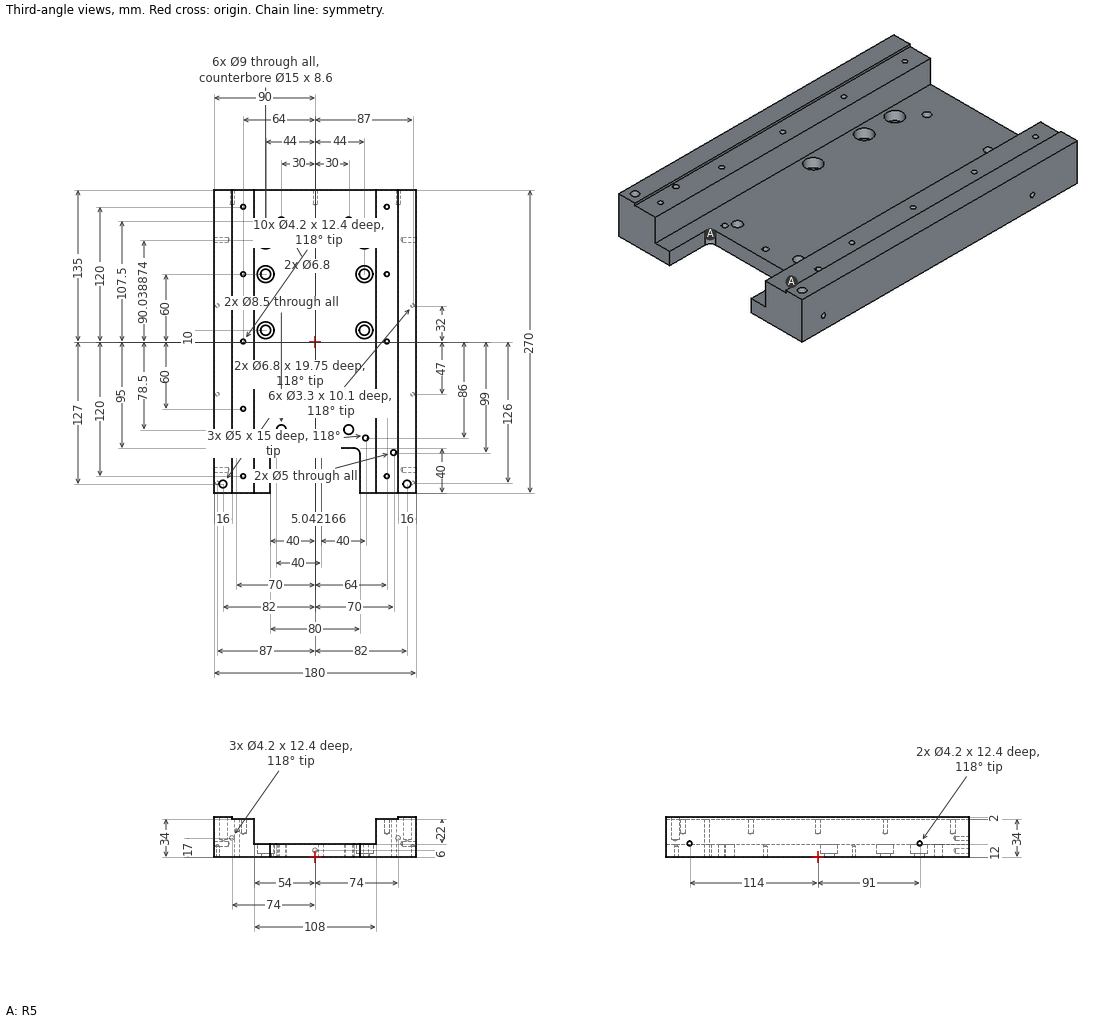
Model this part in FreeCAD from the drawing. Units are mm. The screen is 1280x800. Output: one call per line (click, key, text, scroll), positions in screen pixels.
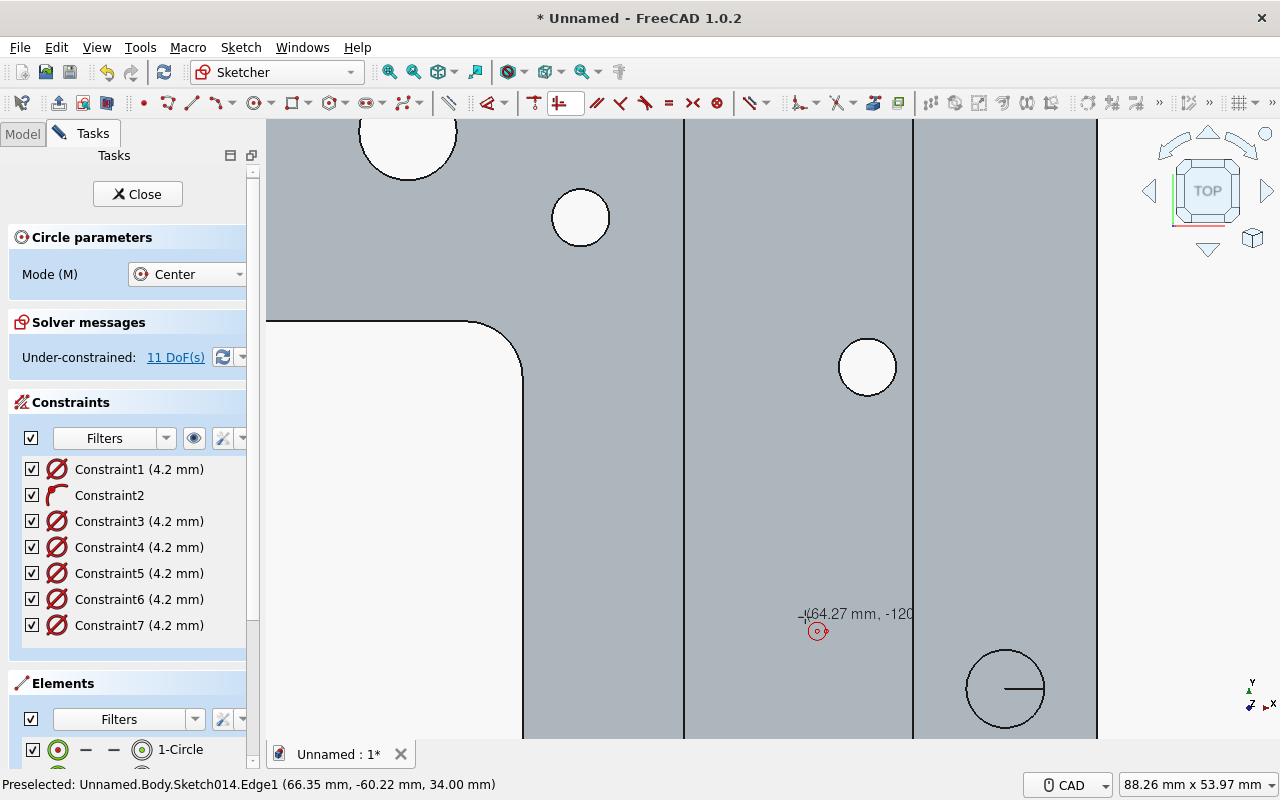
scroll(805, 617, down, 10)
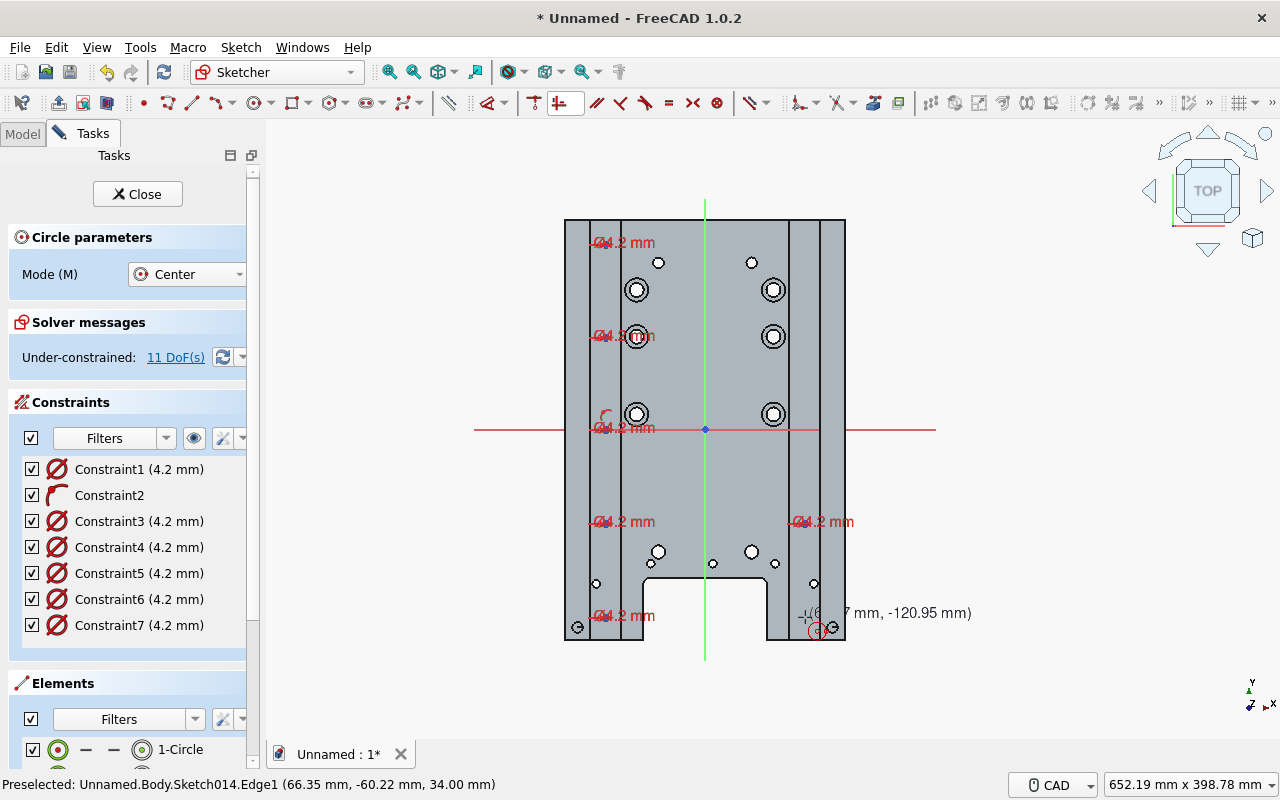
click(805, 617)
move(807, 614)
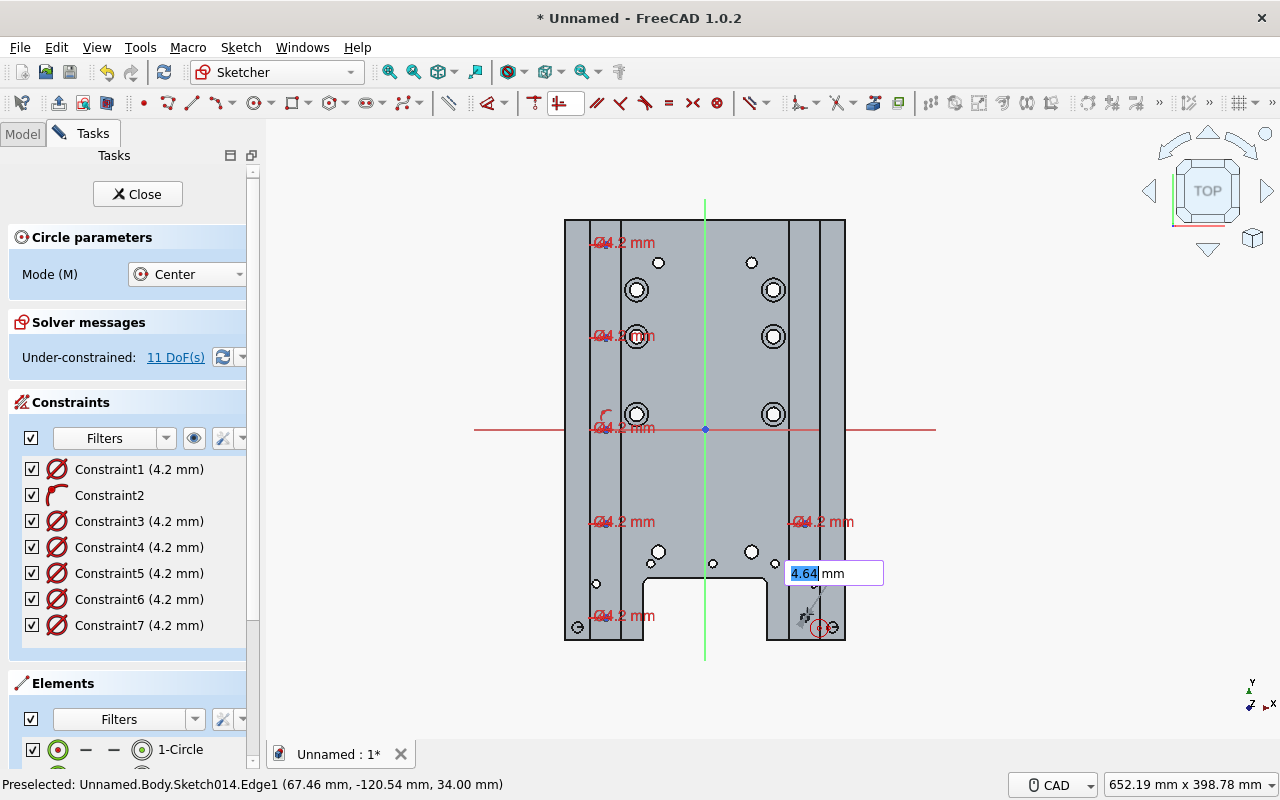
text(4.2)
key(Return)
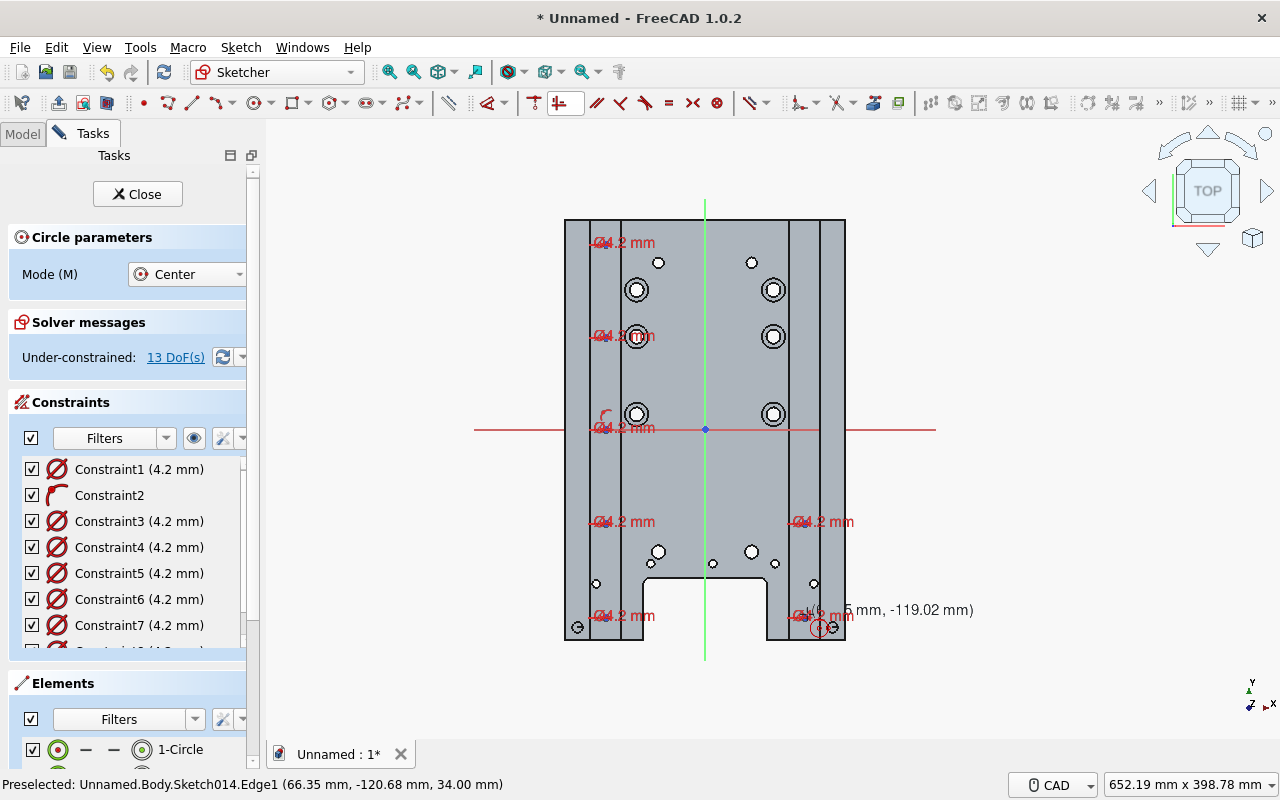
scroll(805, 243, up, 10)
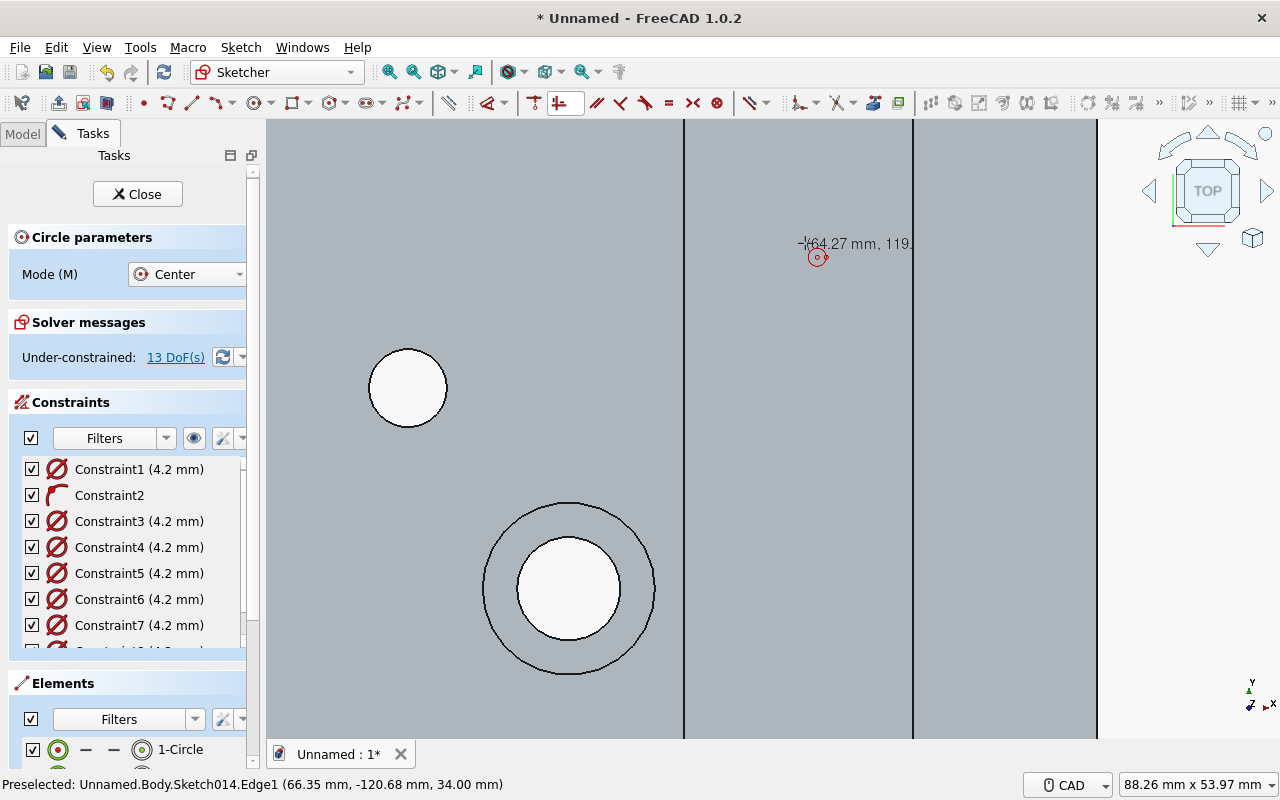
scroll(805, 242, down, 10)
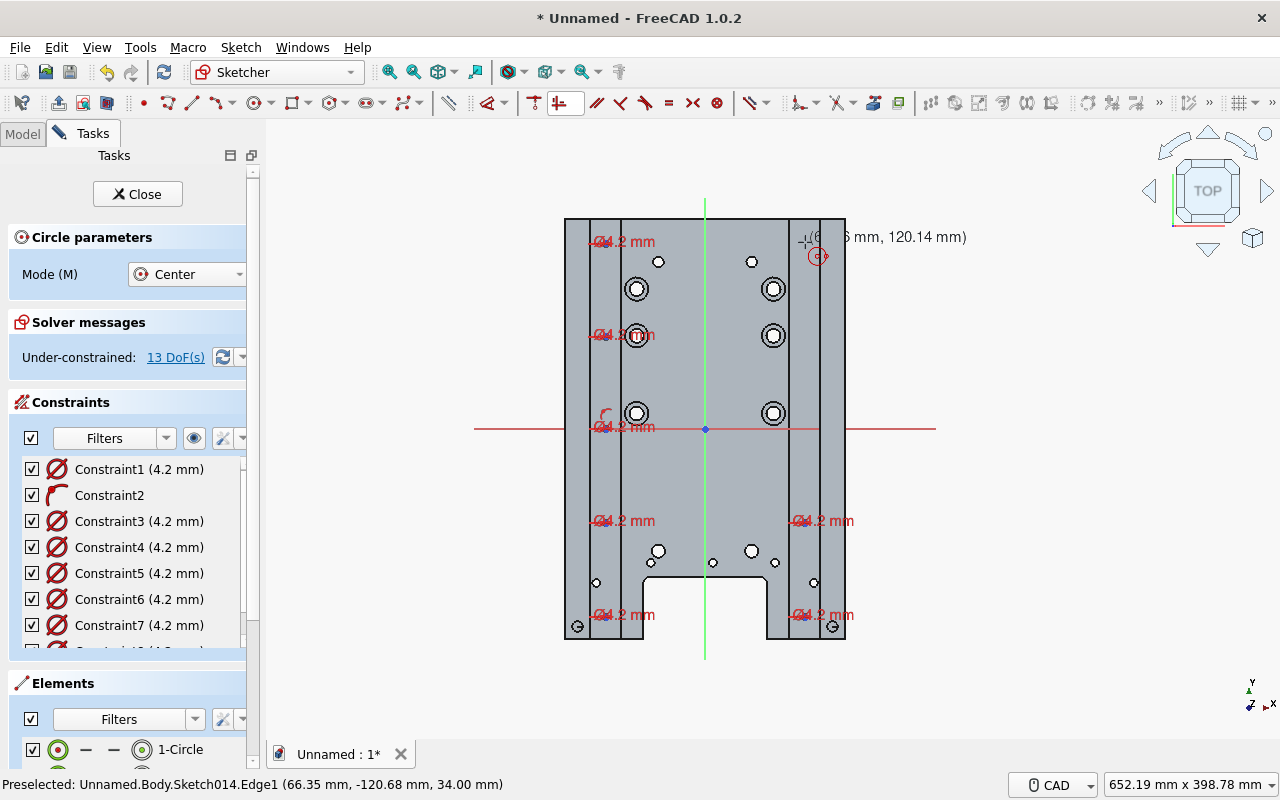
click(805, 243)
move(807, 240)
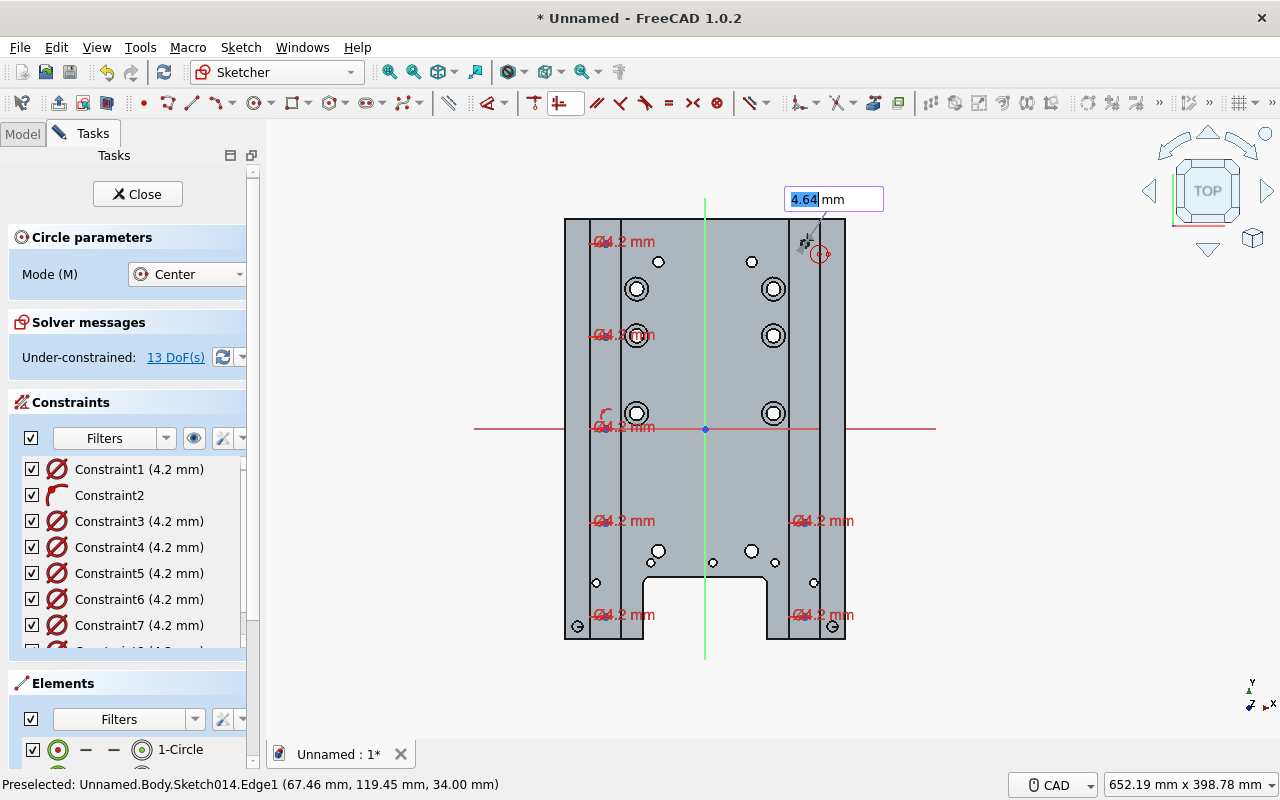
text(4.2)
key(Return)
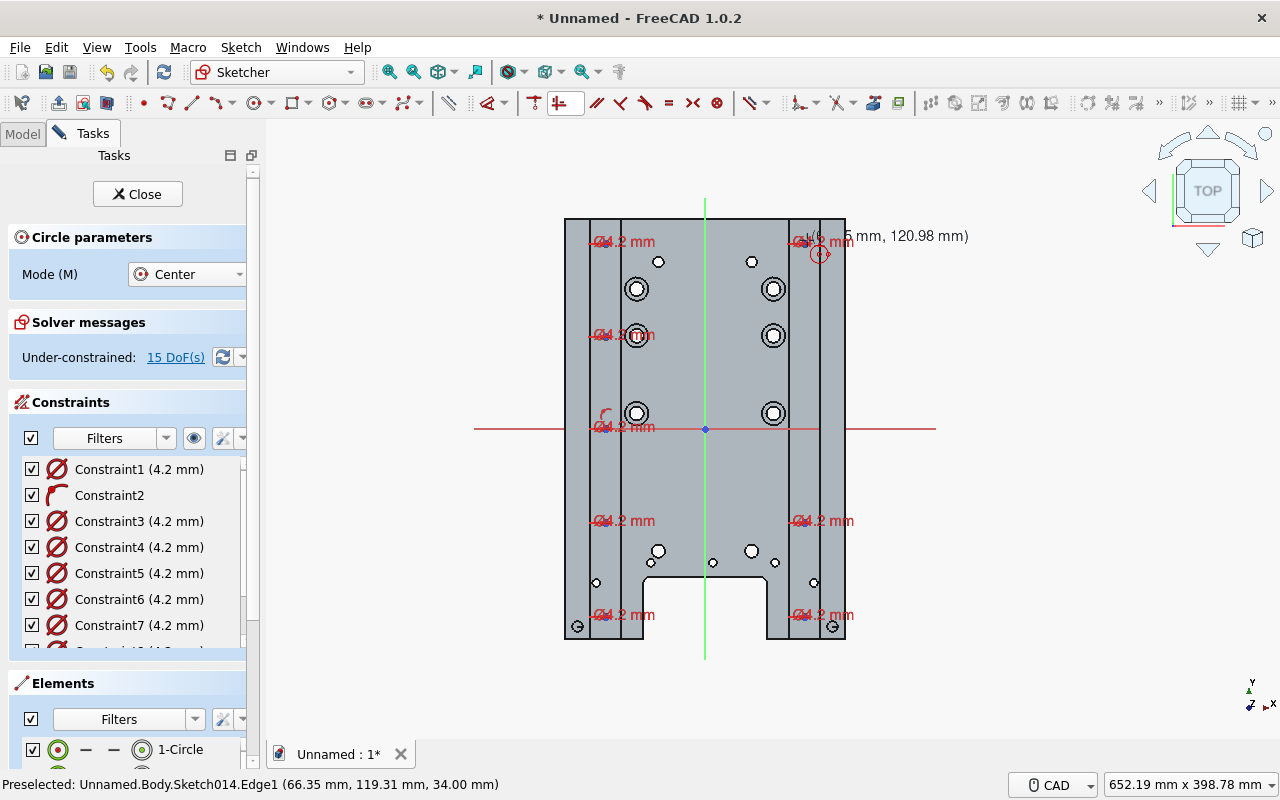
scroll(805, 336, up, 10)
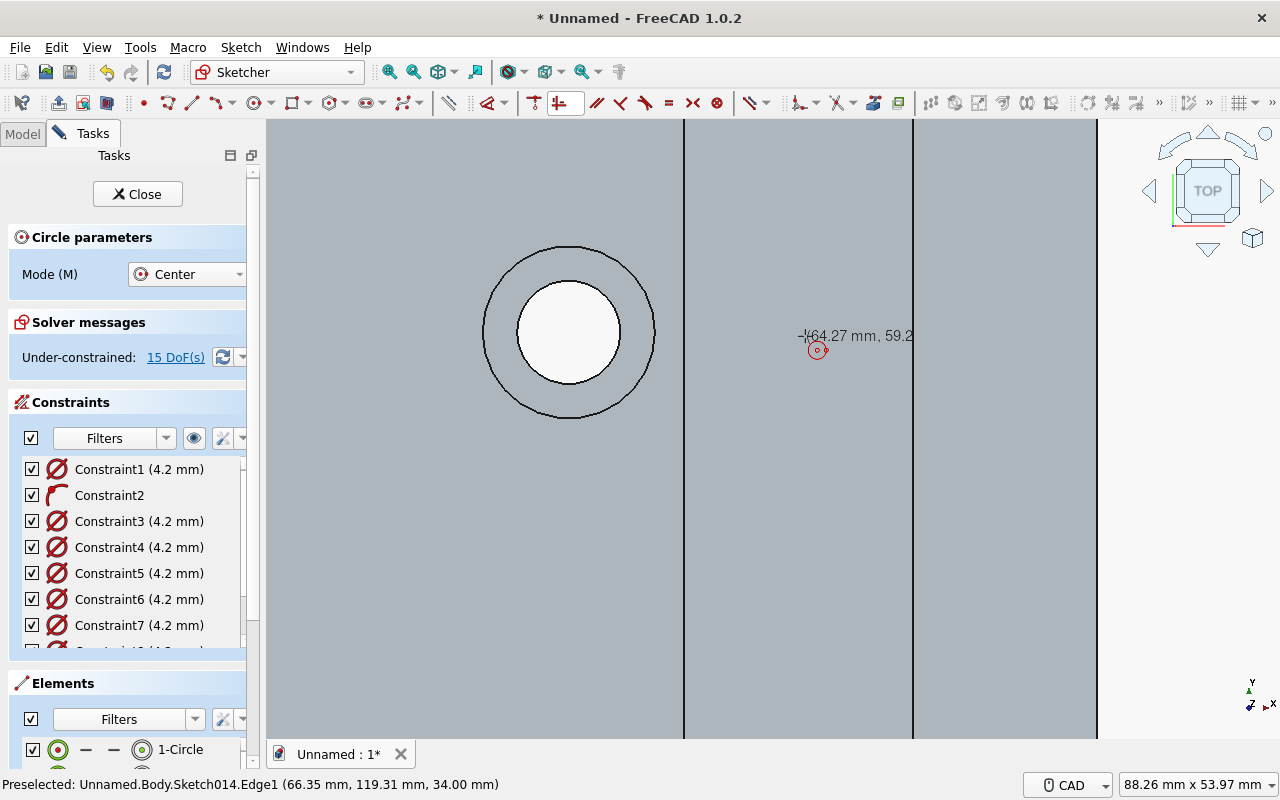
scroll(805, 336, down, 10)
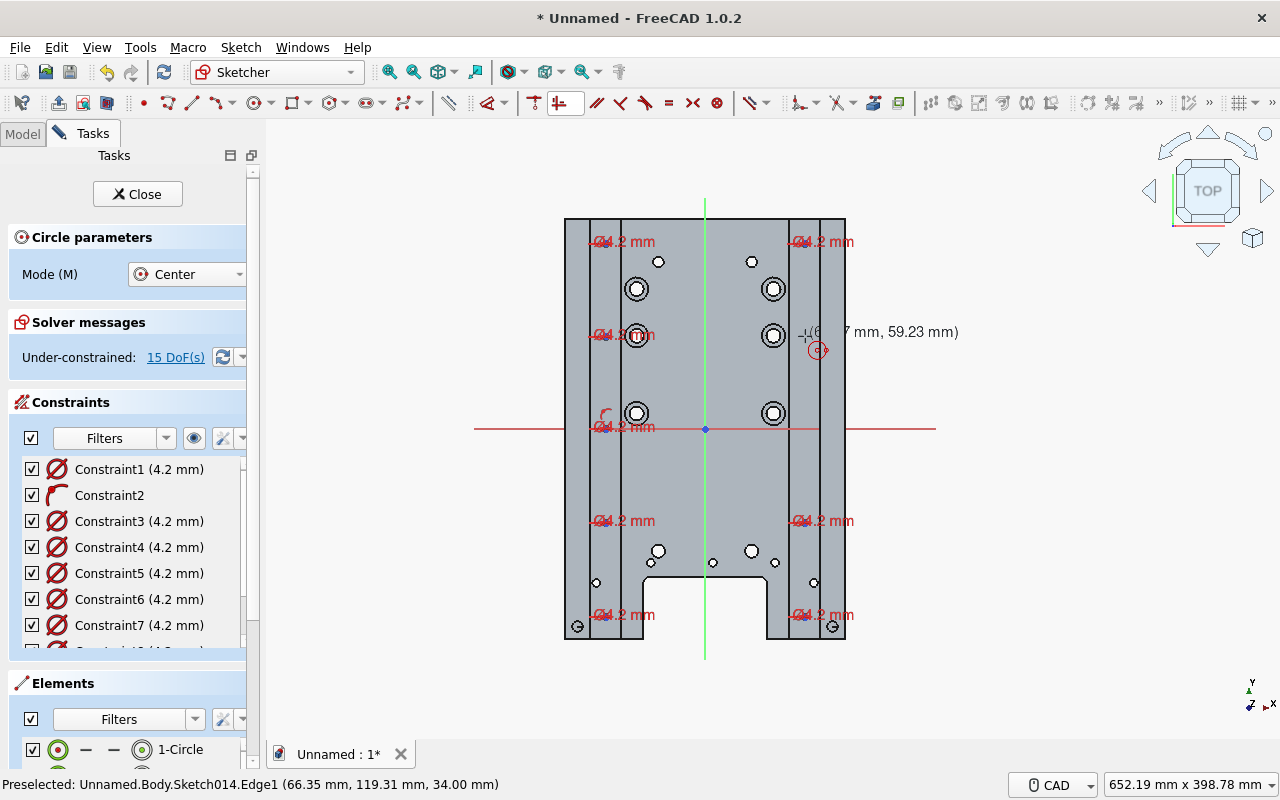
click(805, 336)
move(807, 333)